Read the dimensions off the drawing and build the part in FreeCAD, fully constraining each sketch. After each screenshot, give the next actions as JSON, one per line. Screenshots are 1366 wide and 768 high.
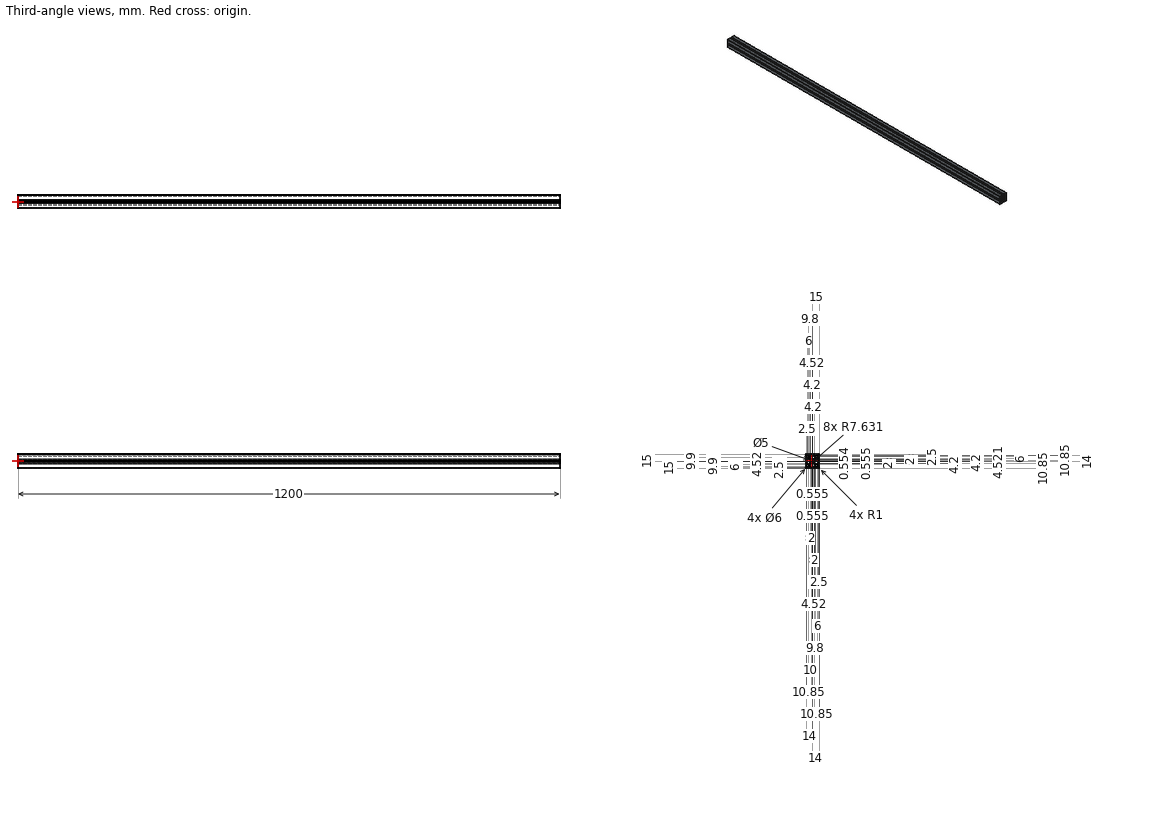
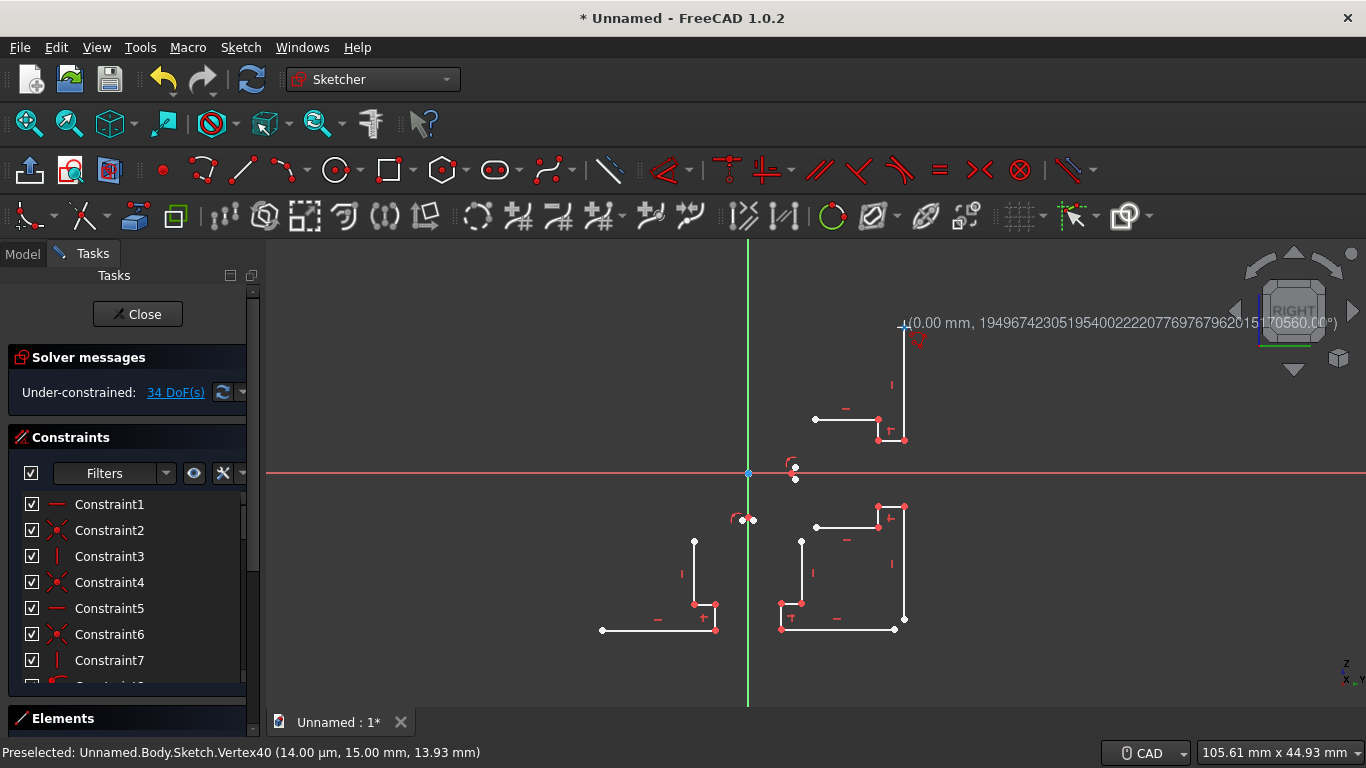
{"action": "left_click", "coordinate": [894, 317]}
{"action": "left_click", "coordinate": [781, 317]}
{"action": "left_click", "coordinate": [781, 343]}
{"action": "left_click", "coordinate": [802, 343]}
{"action": "left_click", "coordinate": [802, 405]}
{"action": "right_click", "coordinate": [802, 405]}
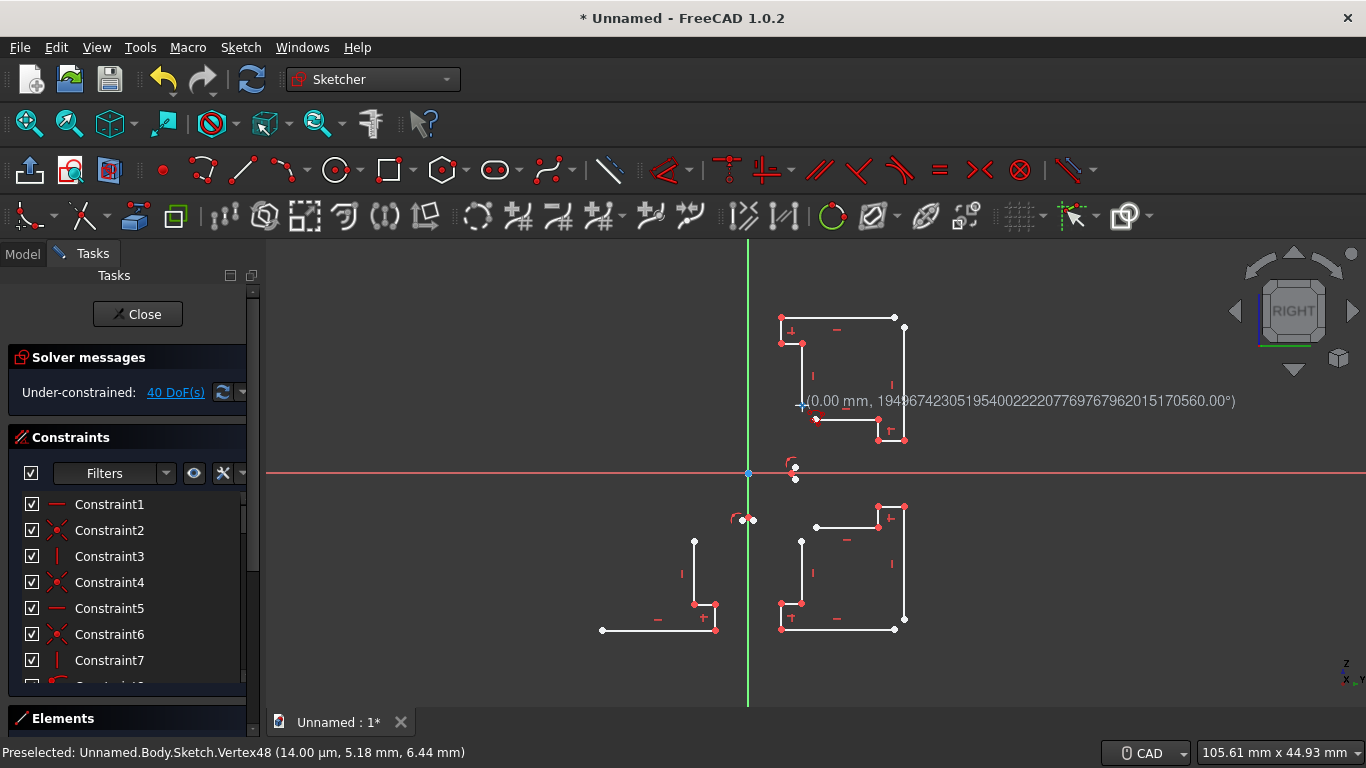
{"action": "scroll", "coordinate": [754, 426], "scroll_direction": "up", "scroll_amount": 6}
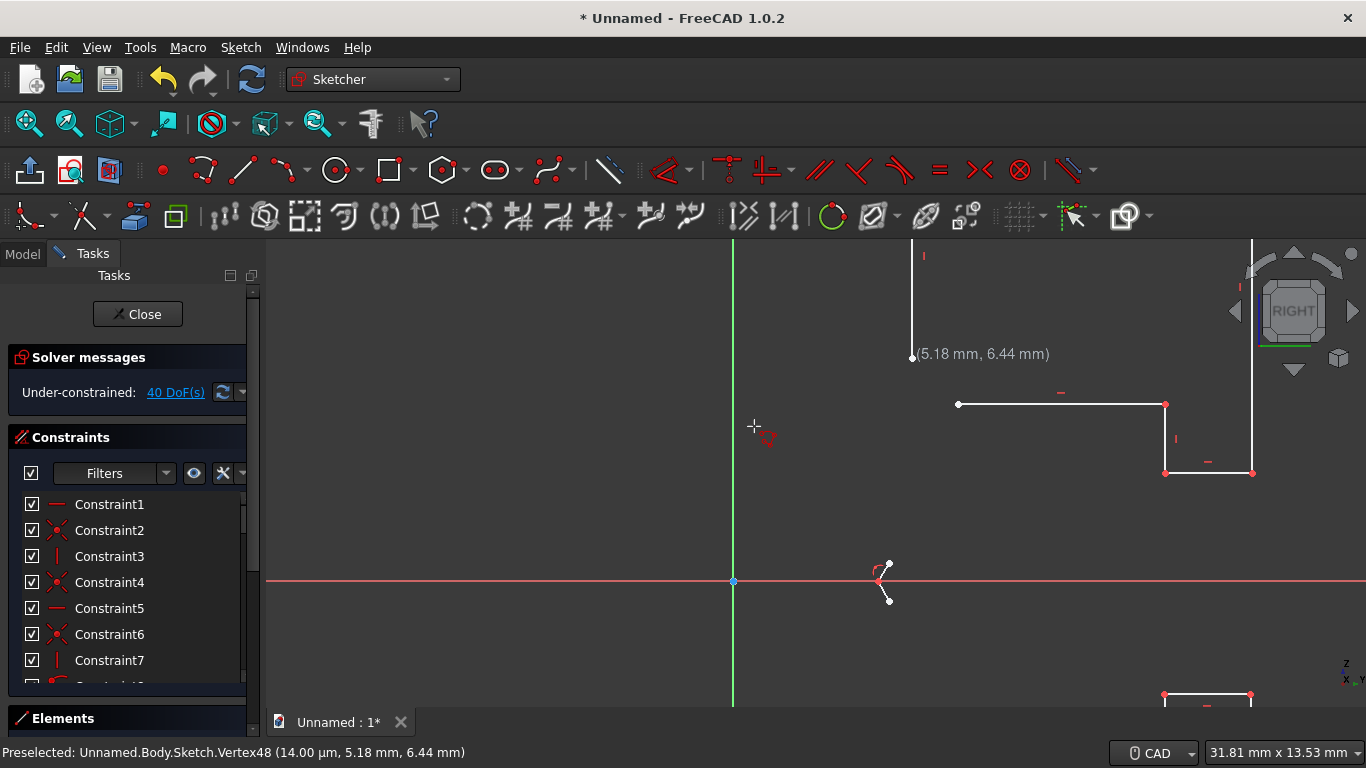
{"action": "left_click", "coordinate": [753, 425]}
{"action": "left_click", "coordinate": [733, 436]}
{"action": "left_click", "coordinate": [714, 425]}
{"action": "right_click", "coordinate": [714, 425]}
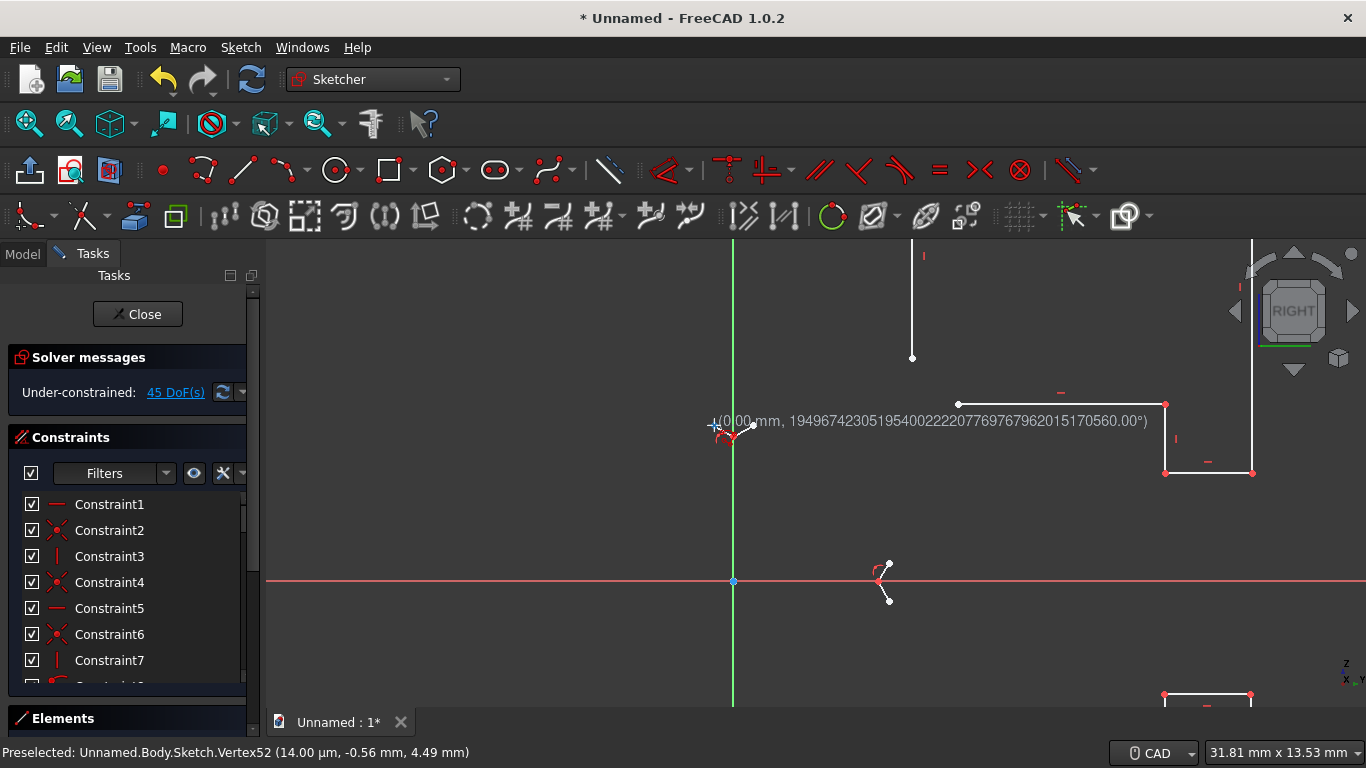
{"action": "left_click", "coordinate": [555, 357]}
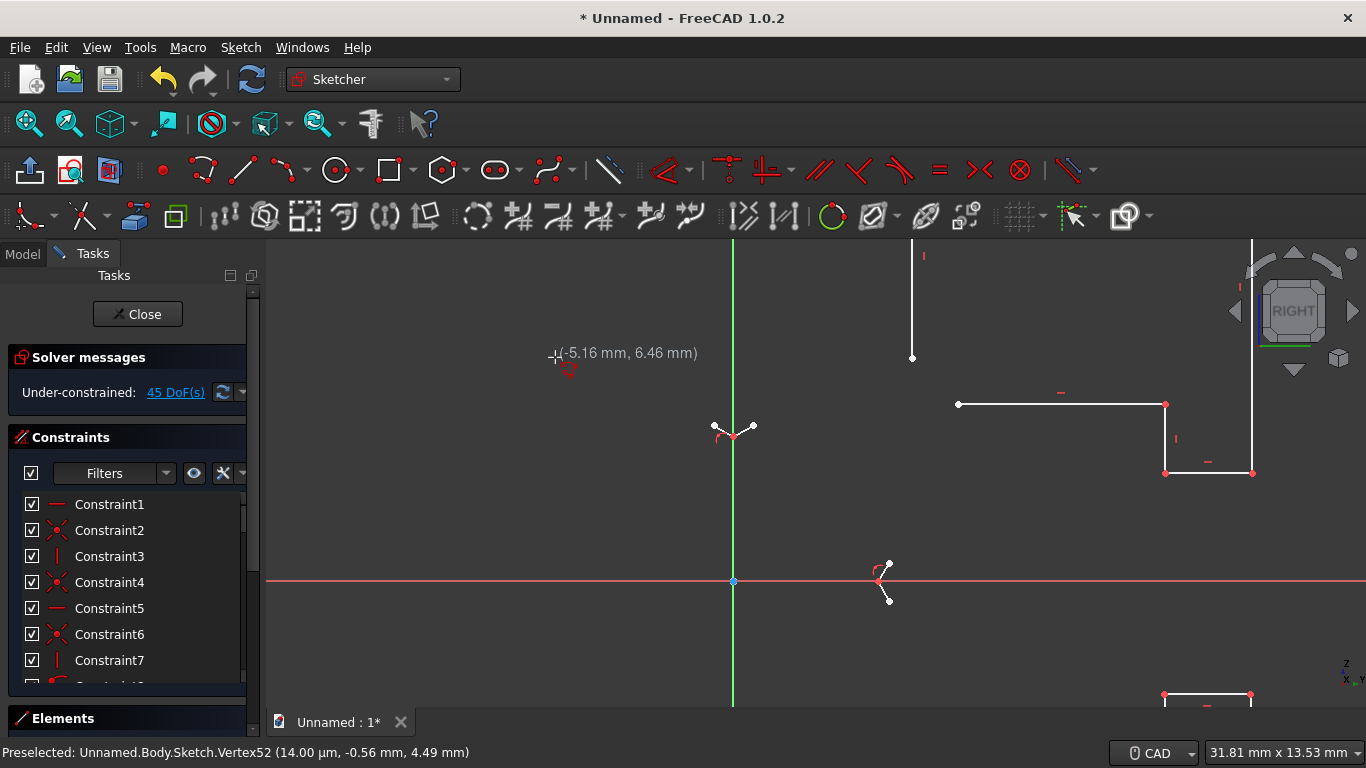
{"action": "scroll", "coordinate": [754, 426], "scroll_direction": "down", "scroll_amount": 6}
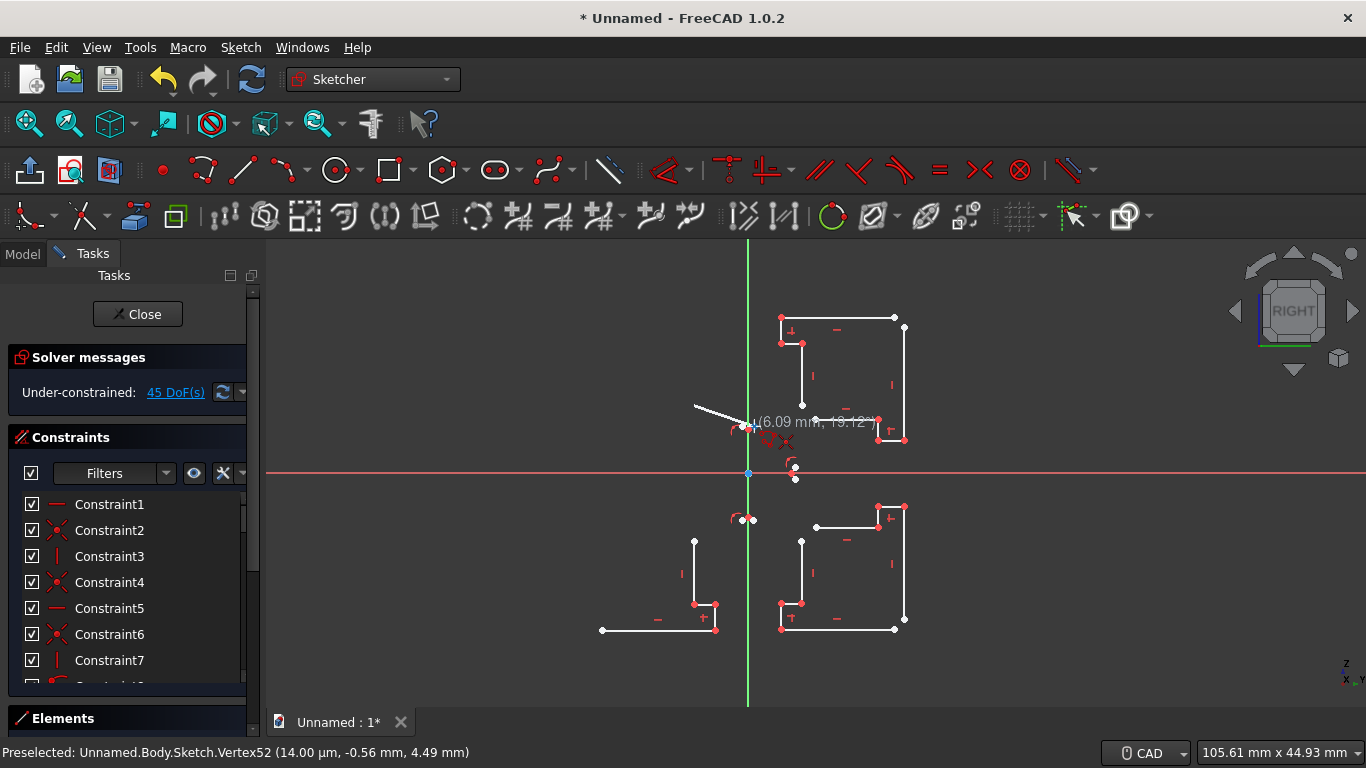
{"action": "left_click", "coordinate": [694, 343]}
{"action": "left_click", "coordinate": [715, 343]}
{"action": "left_click", "coordinate": [715, 317]}
{"action": "left_click", "coordinate": [602, 317]}
{"action": "right_click", "coordinate": [602, 317]}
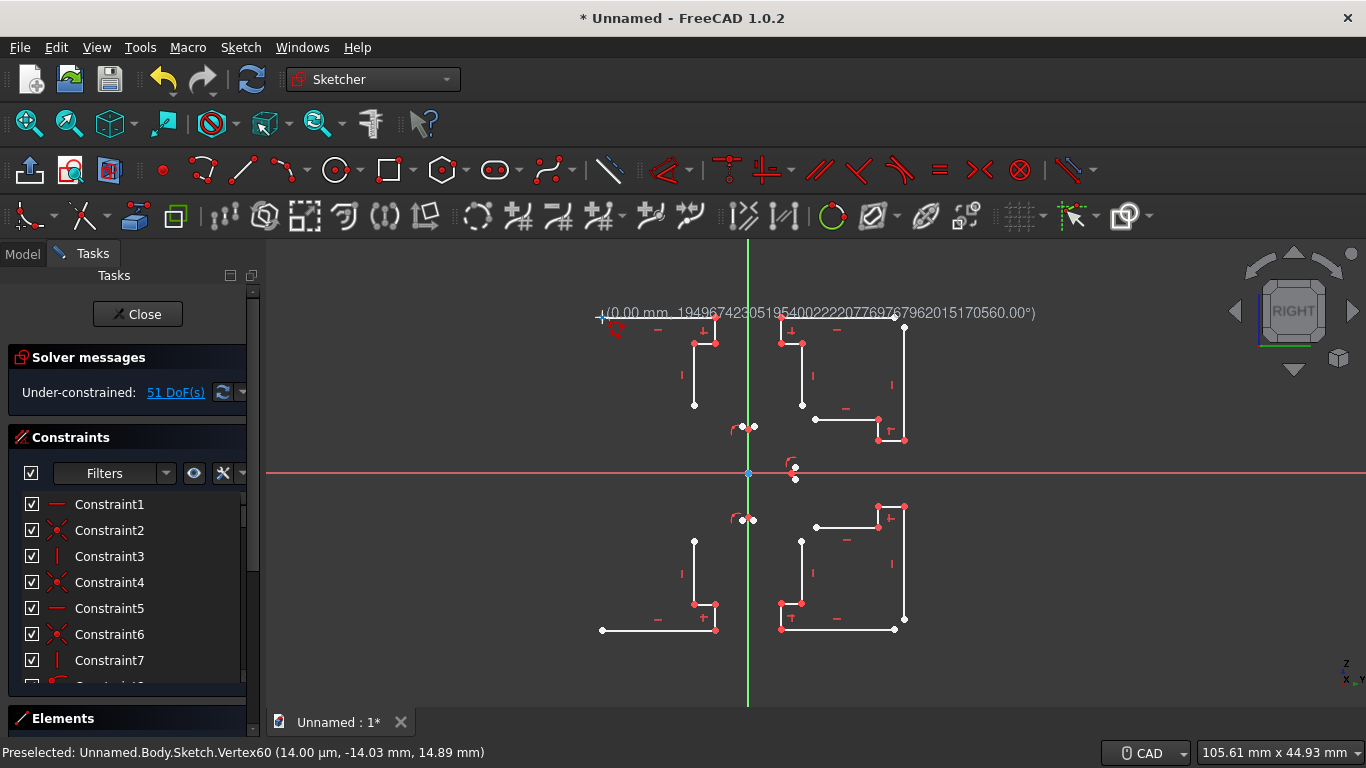
{"action": "left_click", "coordinate": [592, 327]}
{"action": "left_click", "coordinate": [592, 440]}
{"action": "left_click", "coordinate": [618, 440]}
{"action": "left_click", "coordinate": [618, 419]}
{"action": "left_click", "coordinate": [680, 419]}
{"action": "right_click", "coordinate": [680, 419]}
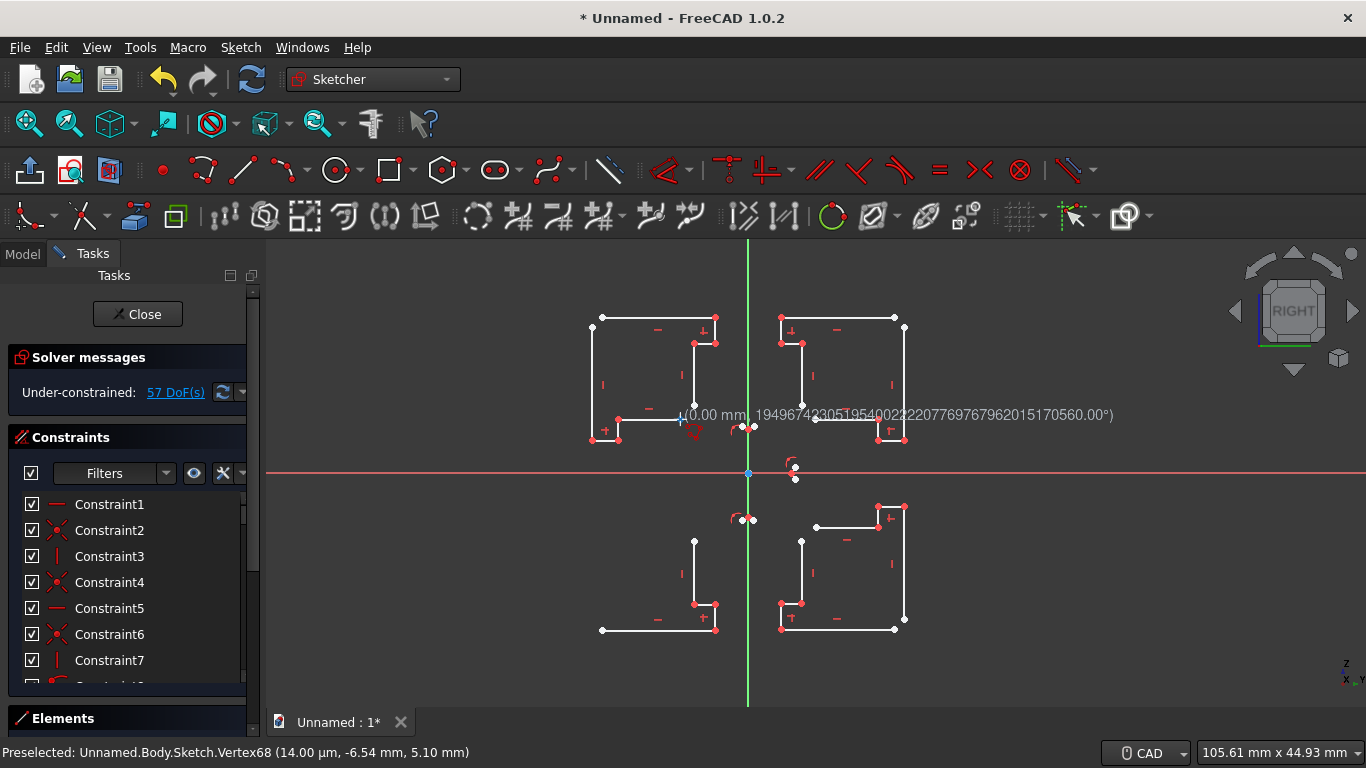
{"action": "scroll", "coordinate": [701, 467], "scroll_direction": "up", "scroll_amount": 6}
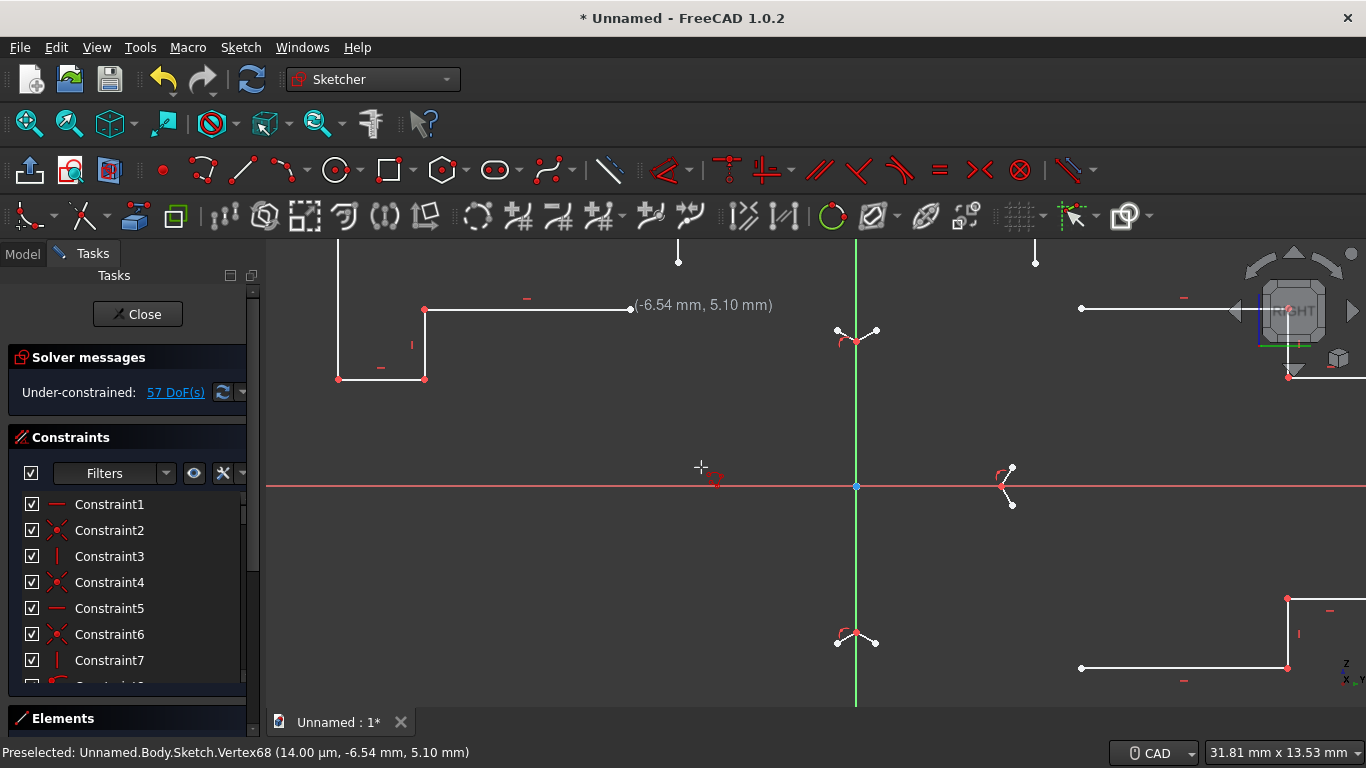
{"action": "left_click", "coordinate": [700, 467]}
{"action": "left_click", "coordinate": [711, 486]}
{"action": "left_click", "coordinate": [700, 505]}
{"action": "right_click", "coordinate": [700, 505]}